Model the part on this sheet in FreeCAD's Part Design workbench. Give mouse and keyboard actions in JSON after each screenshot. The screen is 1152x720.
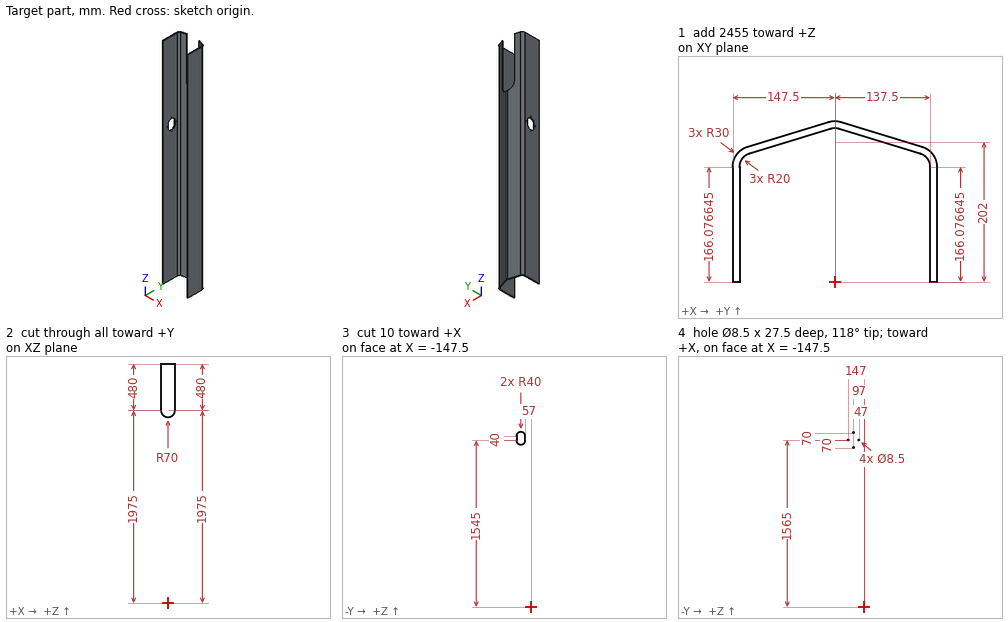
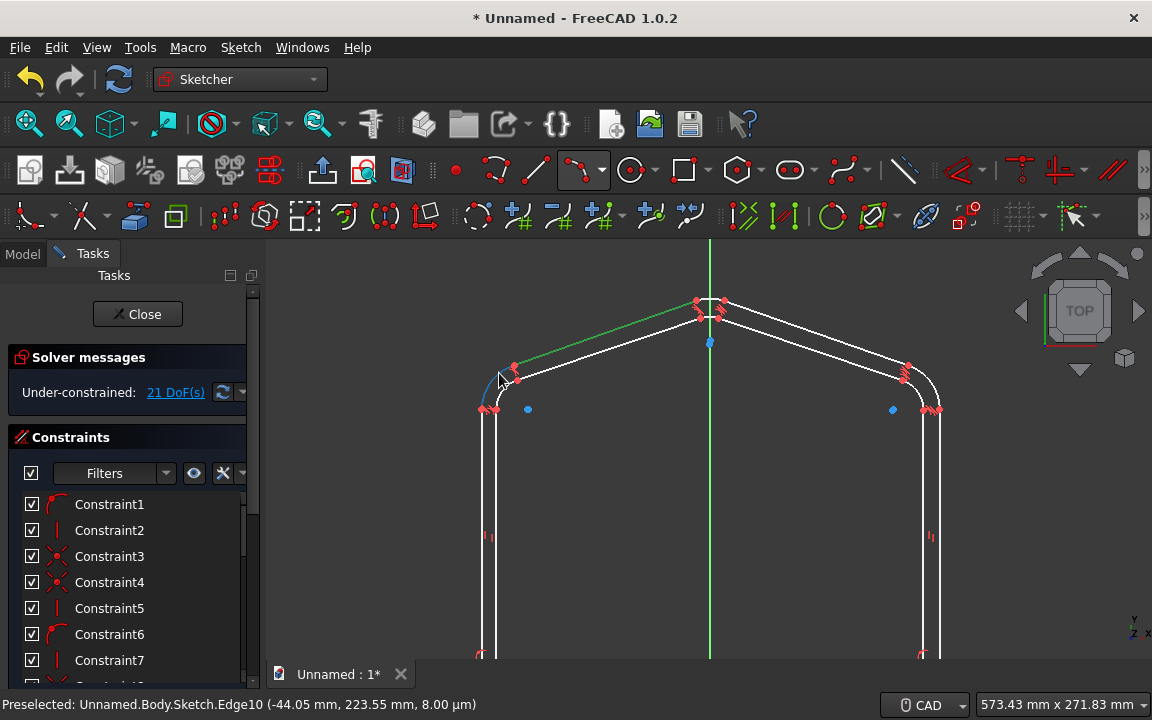
{"action": "left_click", "coordinate": [499, 373]}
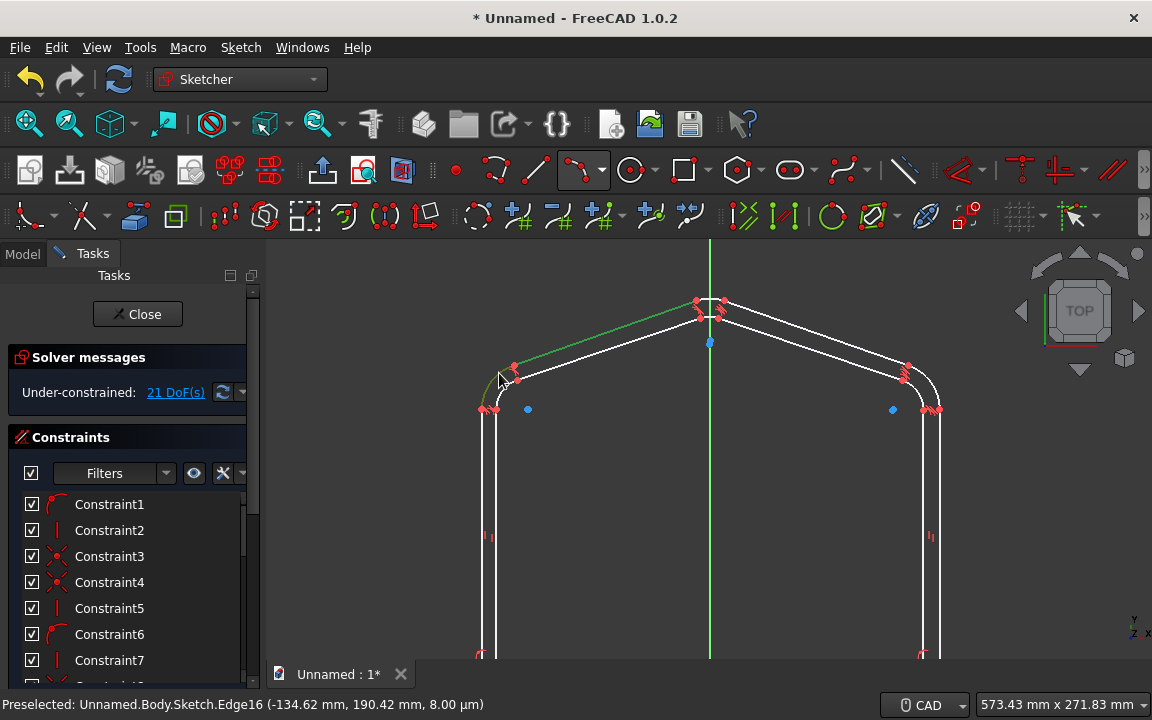
{"action": "key", "text": "t"}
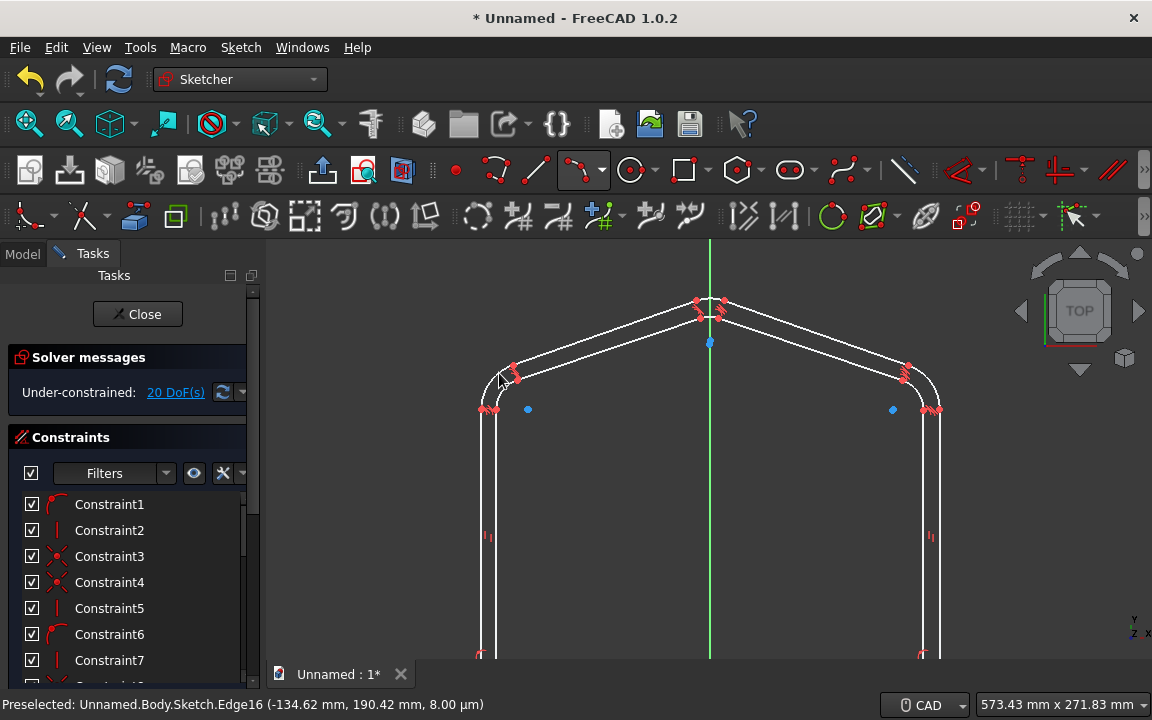
{"action": "scroll", "coordinate": [499, 373], "scroll_direction": "down", "scroll_amount": 2}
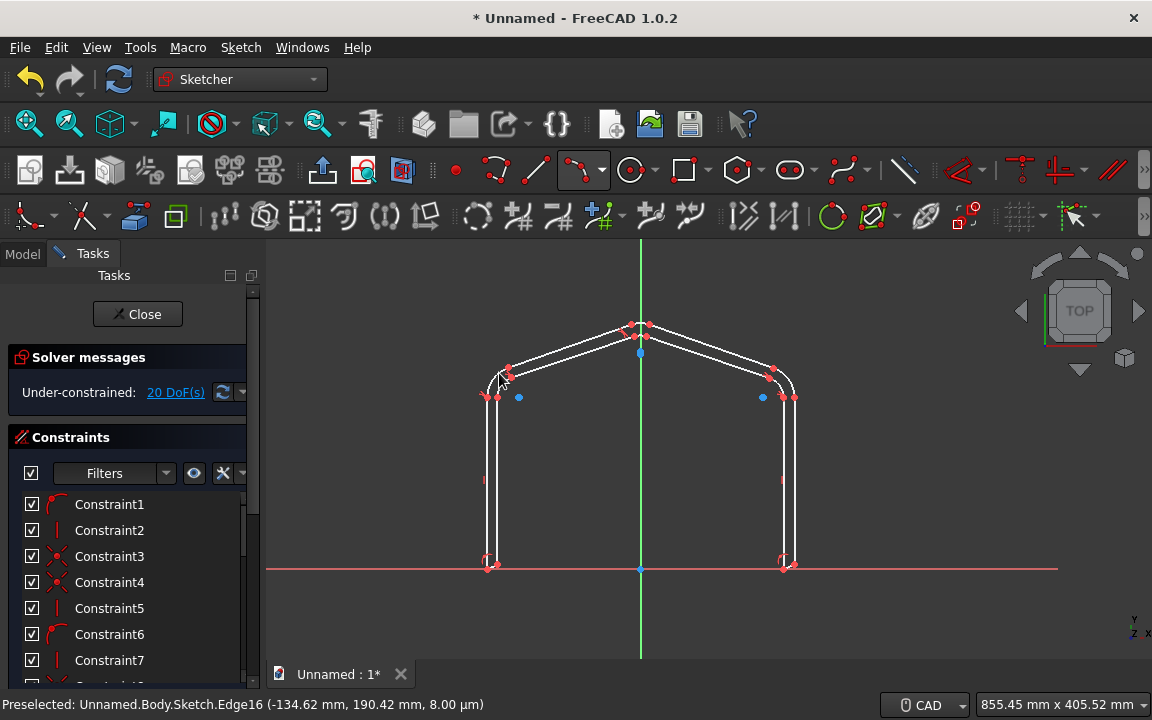
{"action": "scroll", "coordinate": [492, 567], "scroll_direction": "up", "scroll_amount": 6}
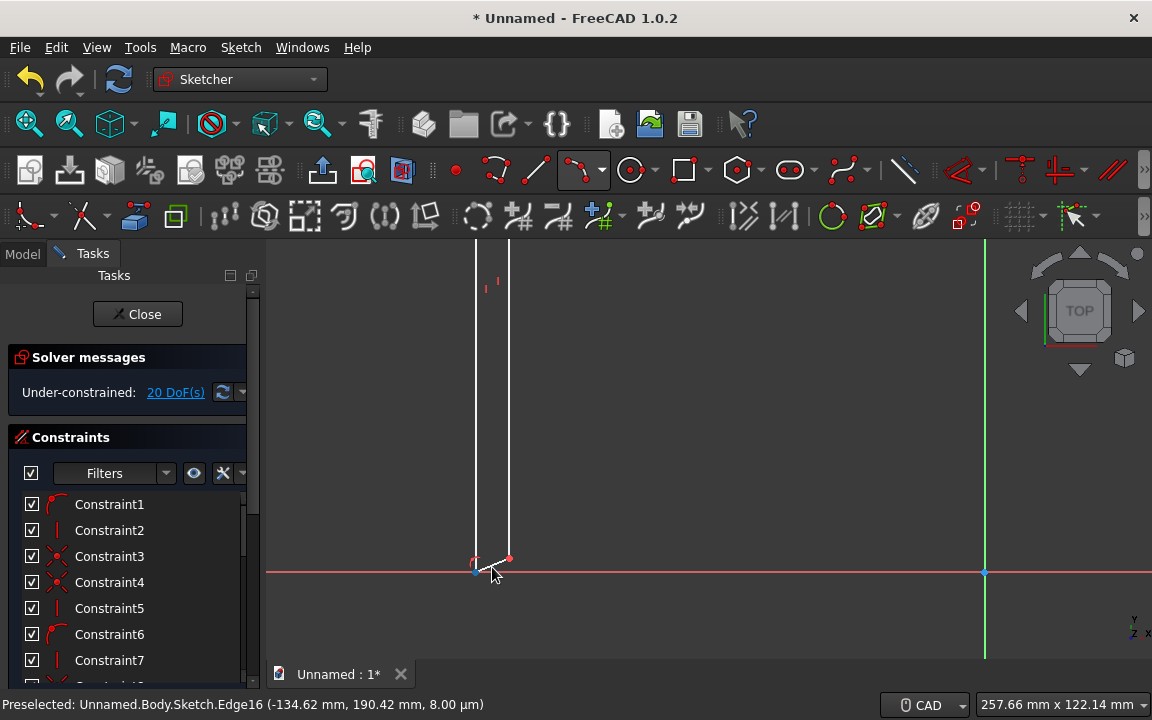
{"action": "left_click", "coordinate": [492, 565]}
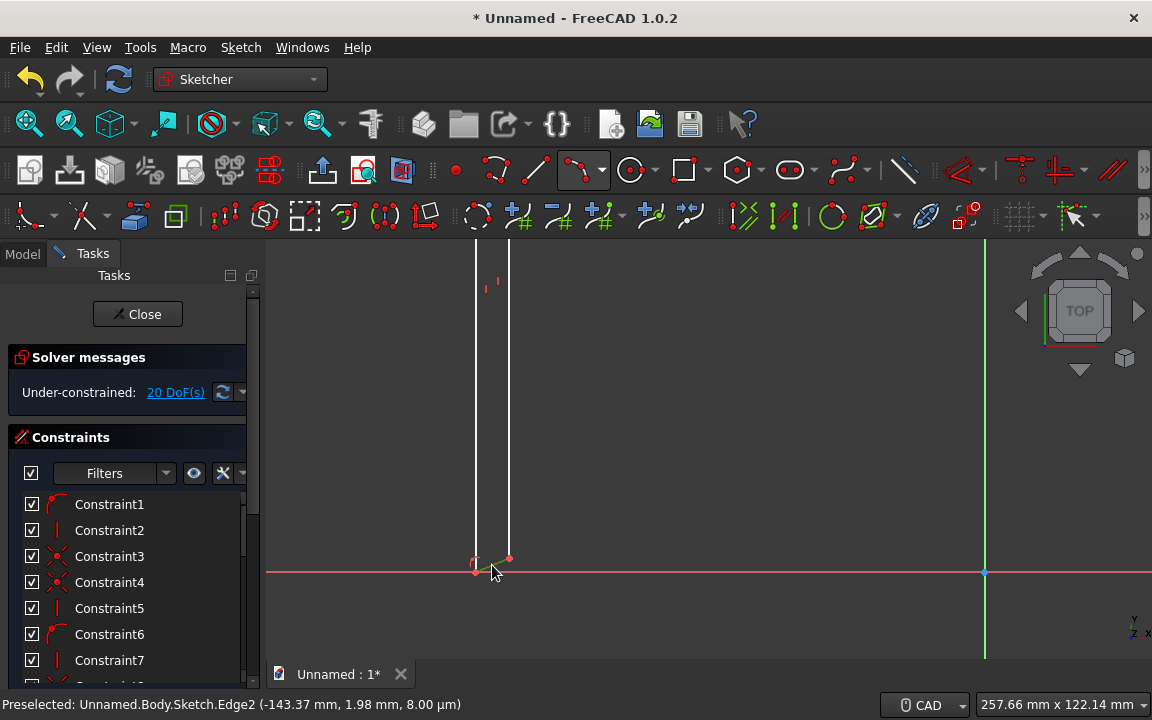
{"action": "left_click", "coordinate": [1086, 170]}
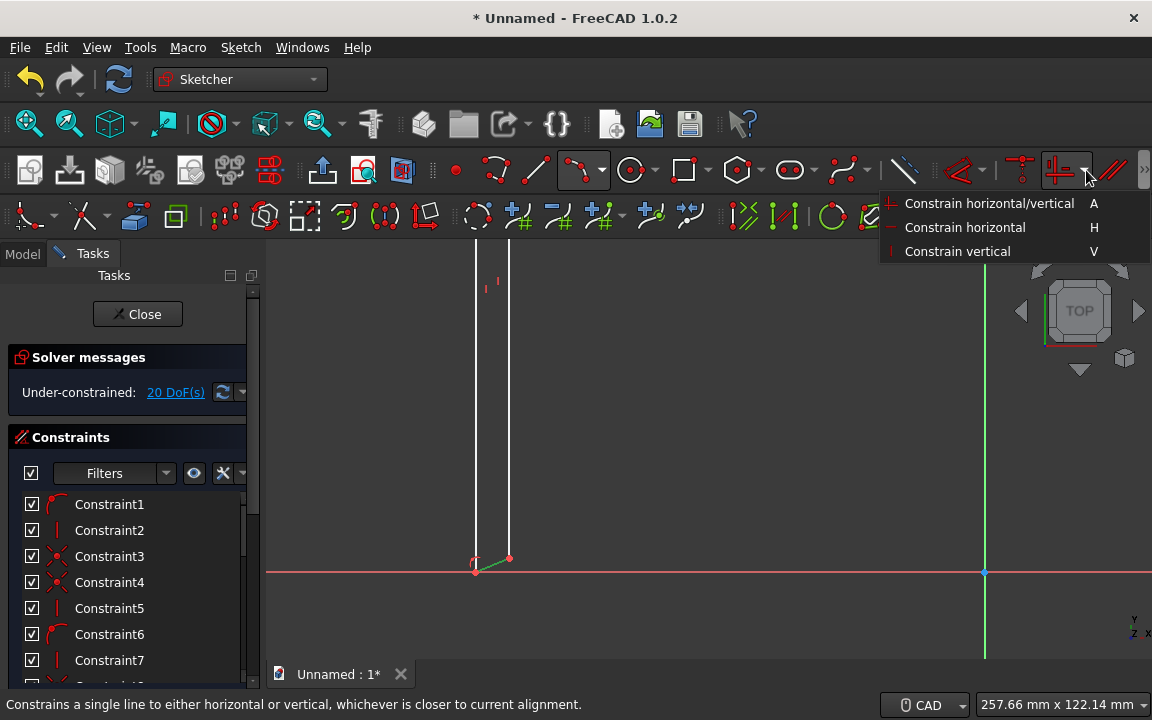
{"action": "left_click", "coordinate": [1015, 227]}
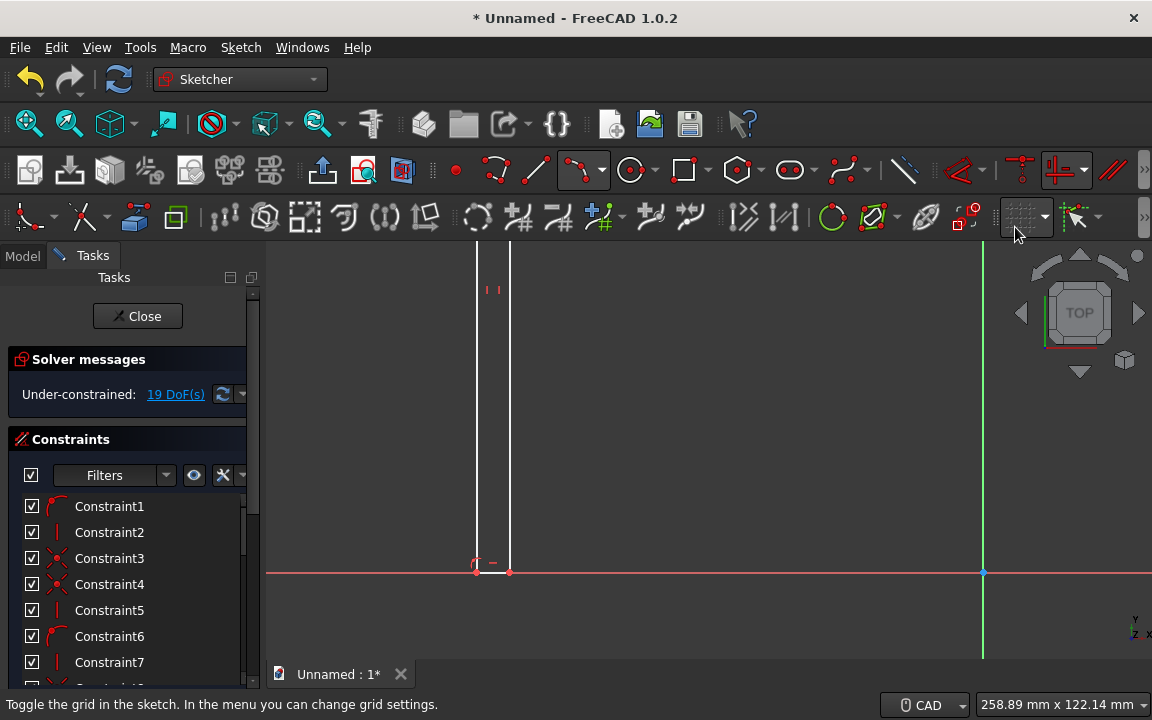
{"action": "scroll", "coordinate": [493, 568], "scroll_direction": "down", "scroll_amount": 6}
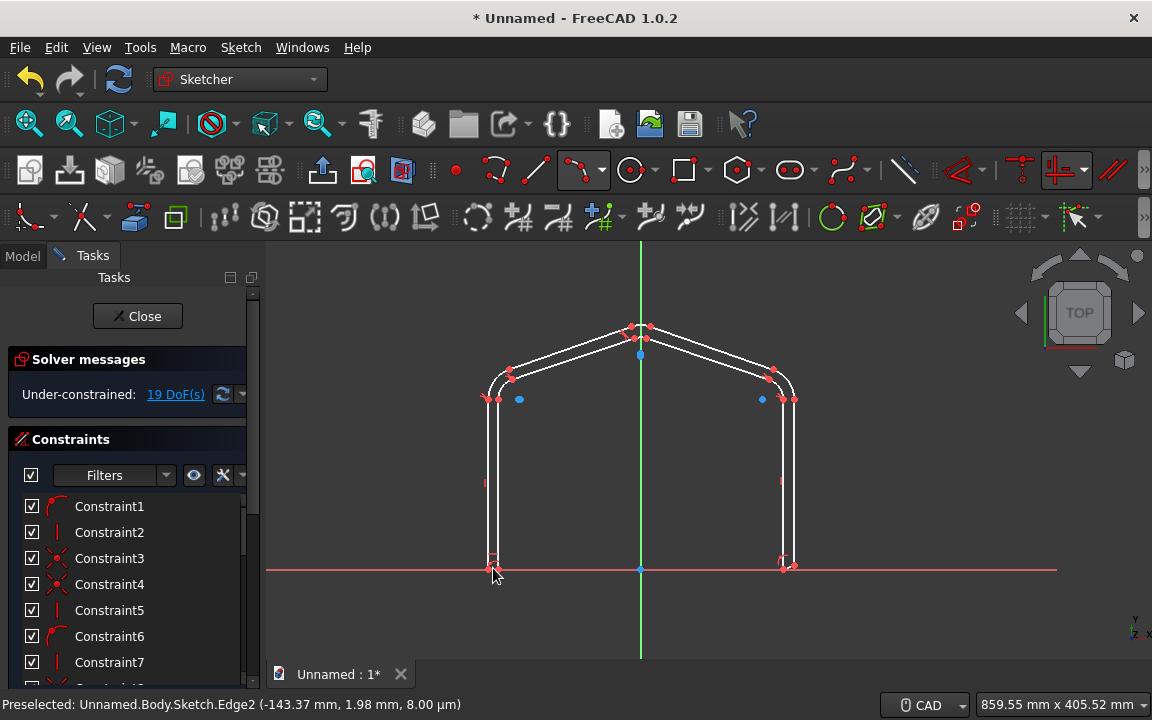
{"action": "scroll", "coordinate": [791, 567], "scroll_direction": "up", "scroll_amount": 8}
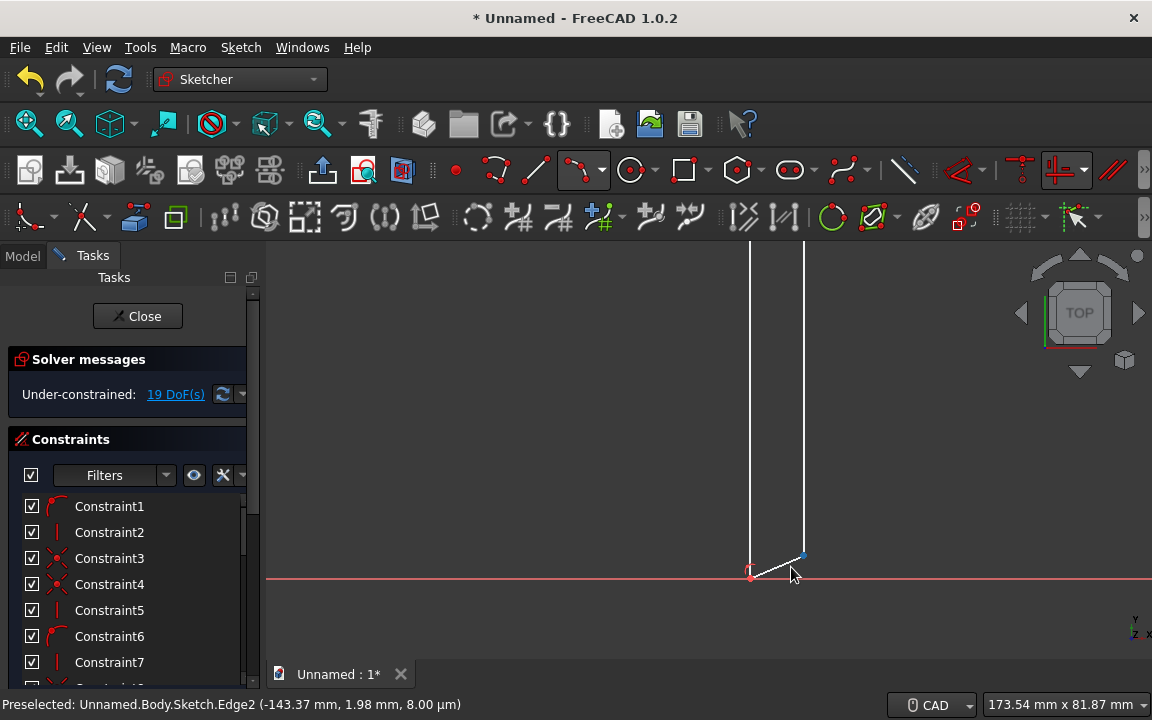
{"action": "left_click", "coordinate": [788, 563]}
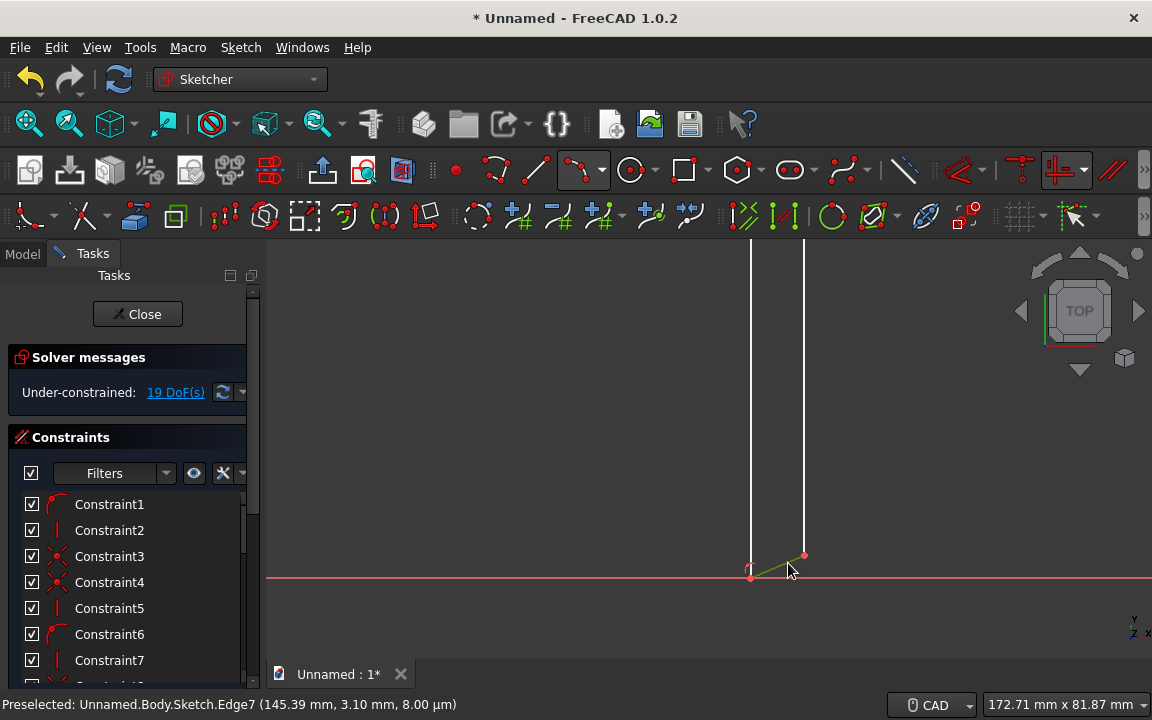
{"action": "left_click", "coordinate": [1086, 170]}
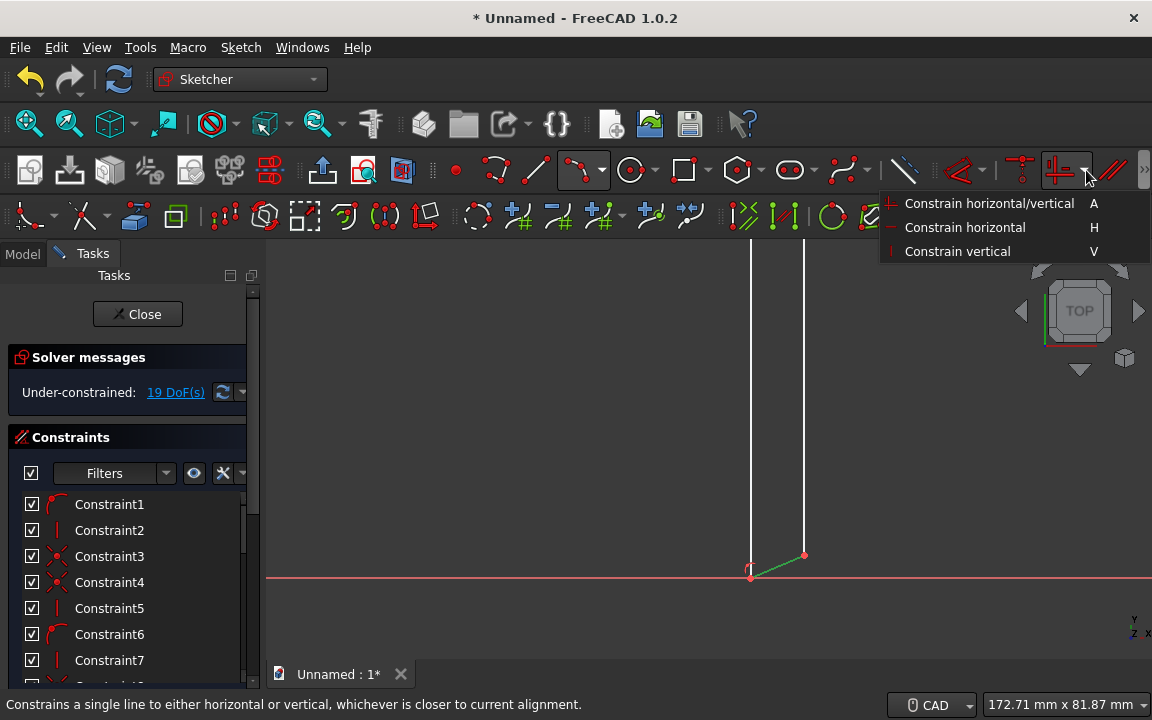
{"action": "left_click", "coordinate": [1015, 227]}